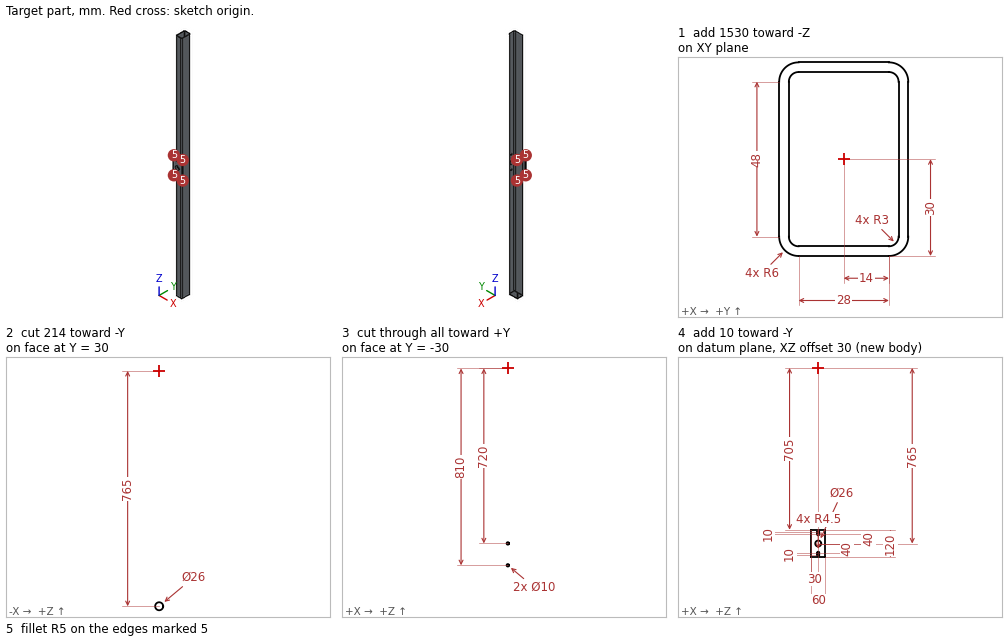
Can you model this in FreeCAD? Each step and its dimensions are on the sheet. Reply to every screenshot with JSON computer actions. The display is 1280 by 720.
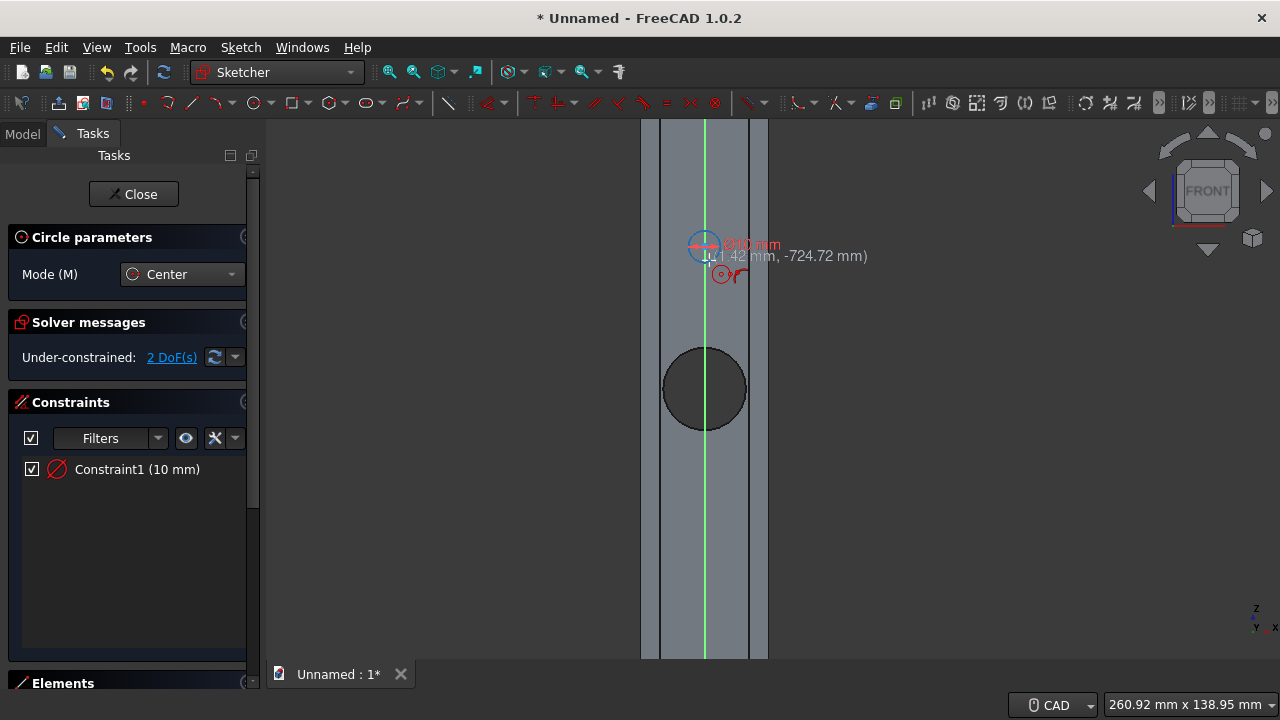
{"action": "scroll", "coordinate": [705, 532], "scroll_direction": "up", "scroll_amount": 2}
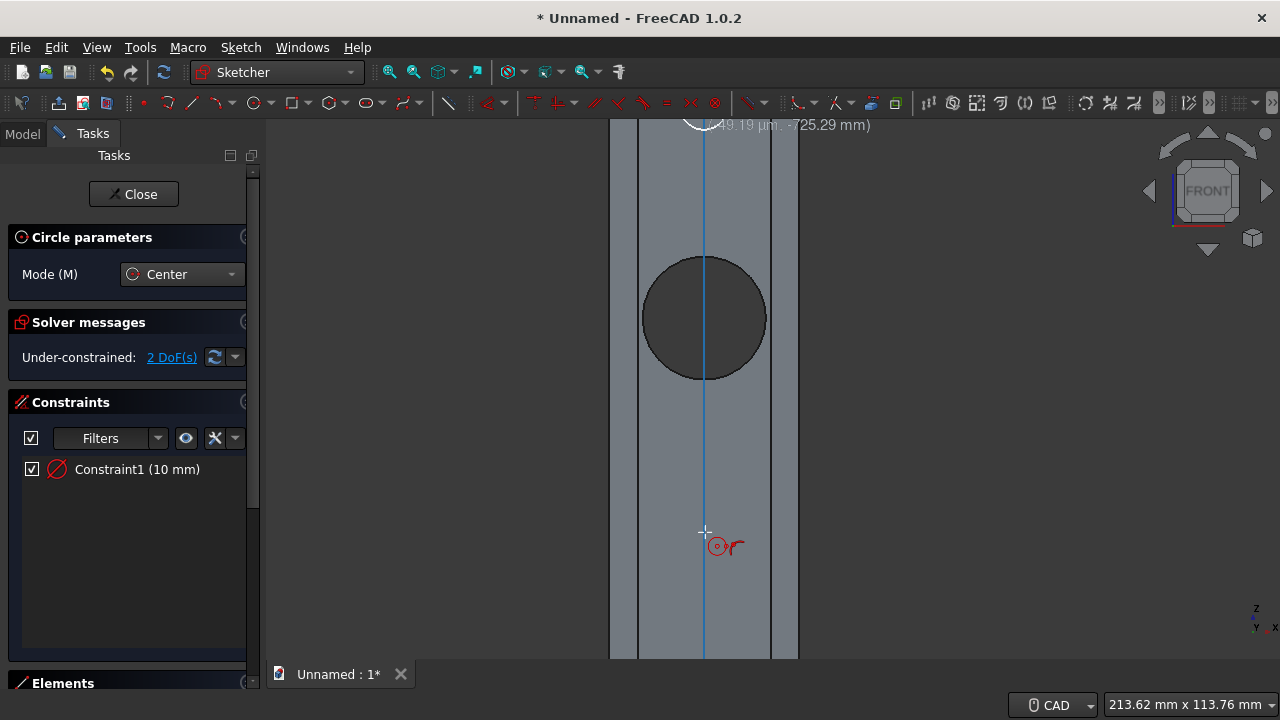
{"action": "left_click", "coordinate": [704, 532]}
{"action": "mouse_move", "coordinate": [721, 515]}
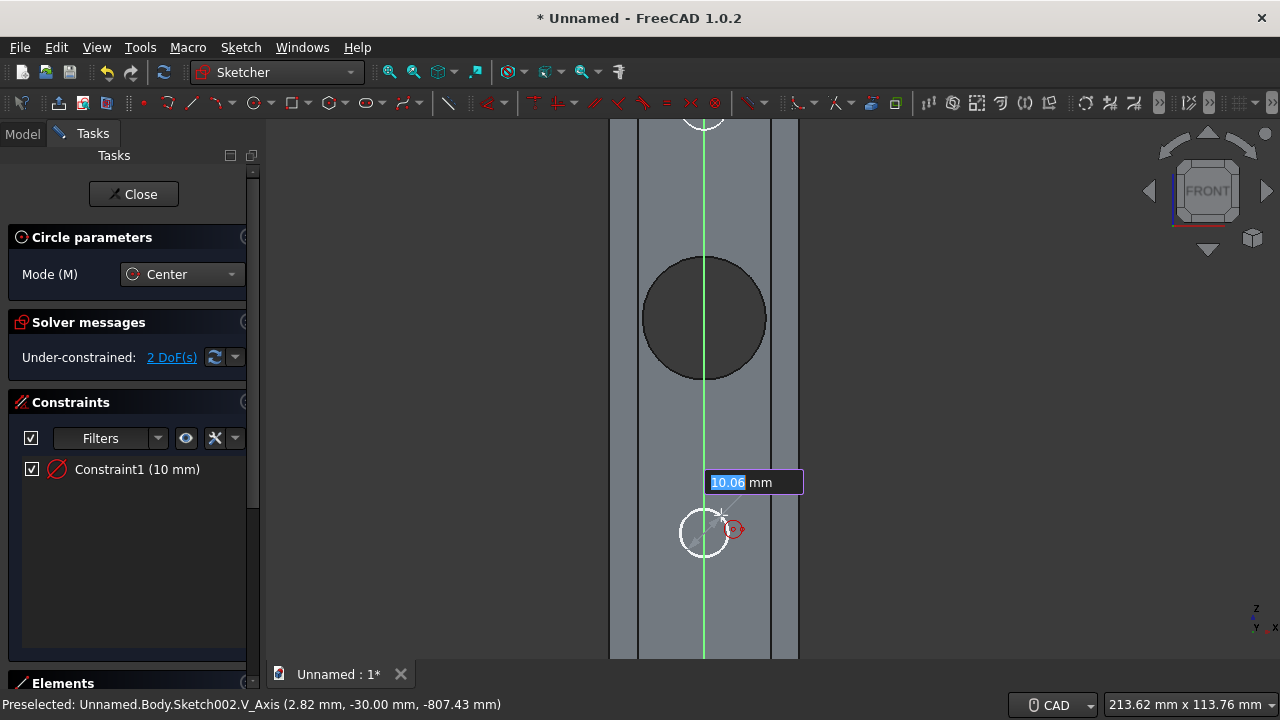
{"action": "type", "text": "10"}
{"action": "key", "text": "Return"}
{"action": "key", "text": "Escape"}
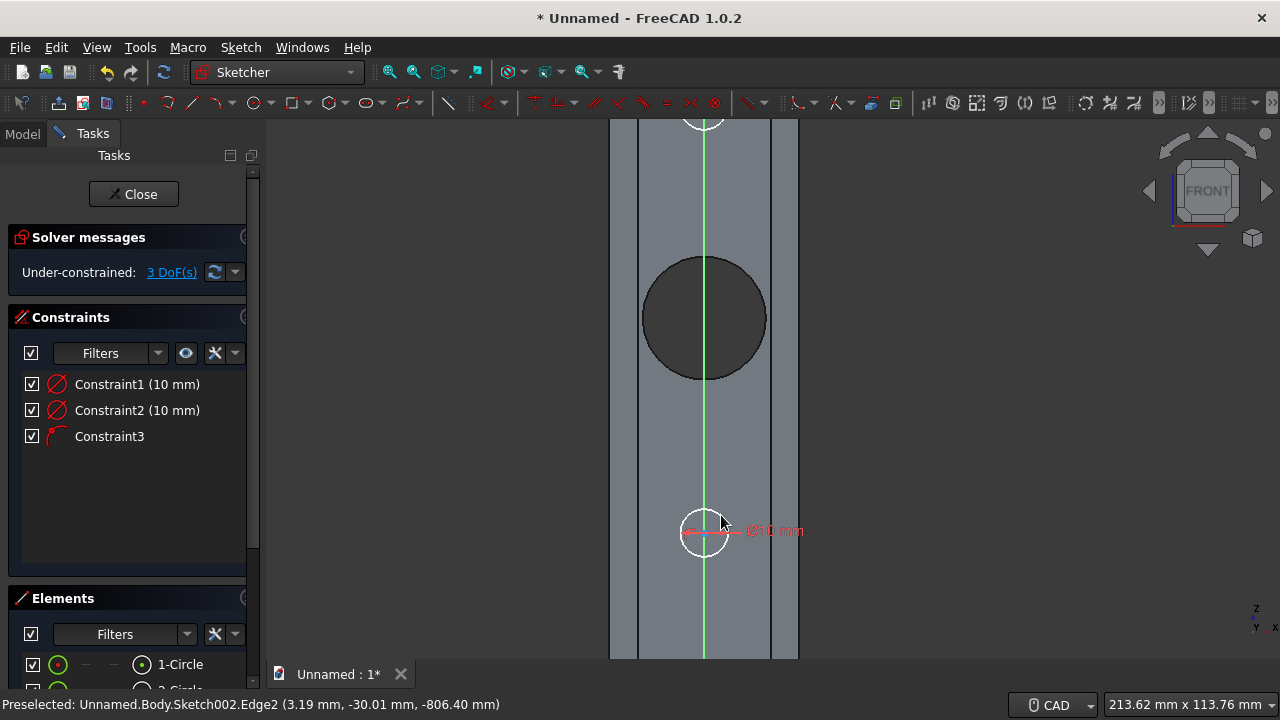
{"action": "scroll", "coordinate": [705, 533], "scroll_direction": "down", "scroll_amount": 2}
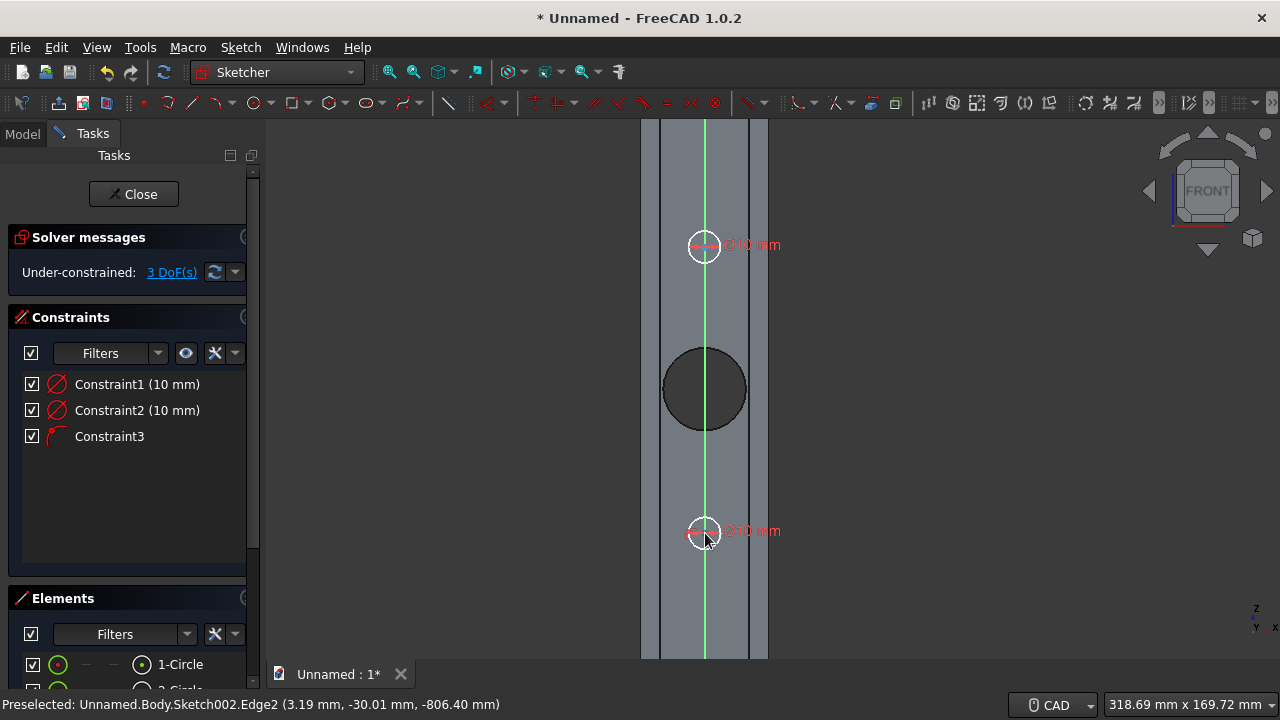
{"action": "left_click", "coordinate": [704, 247]}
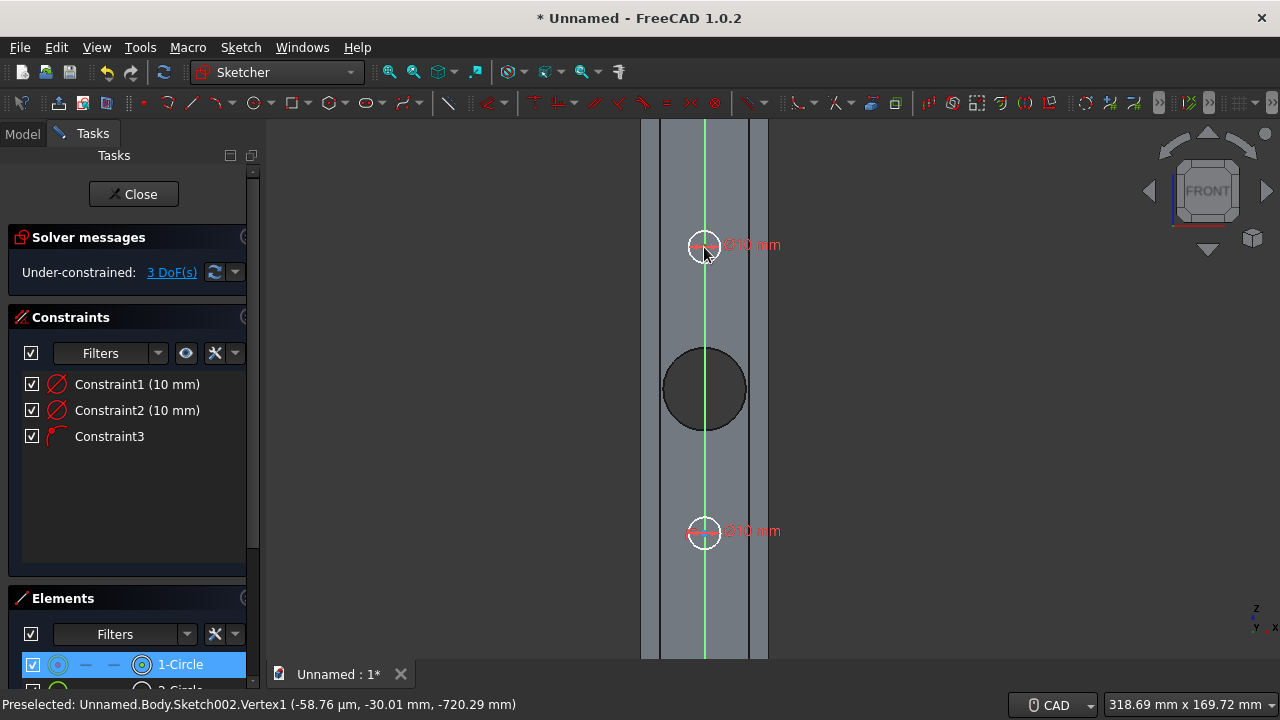
{"action": "left_click", "coordinate": [705, 596]}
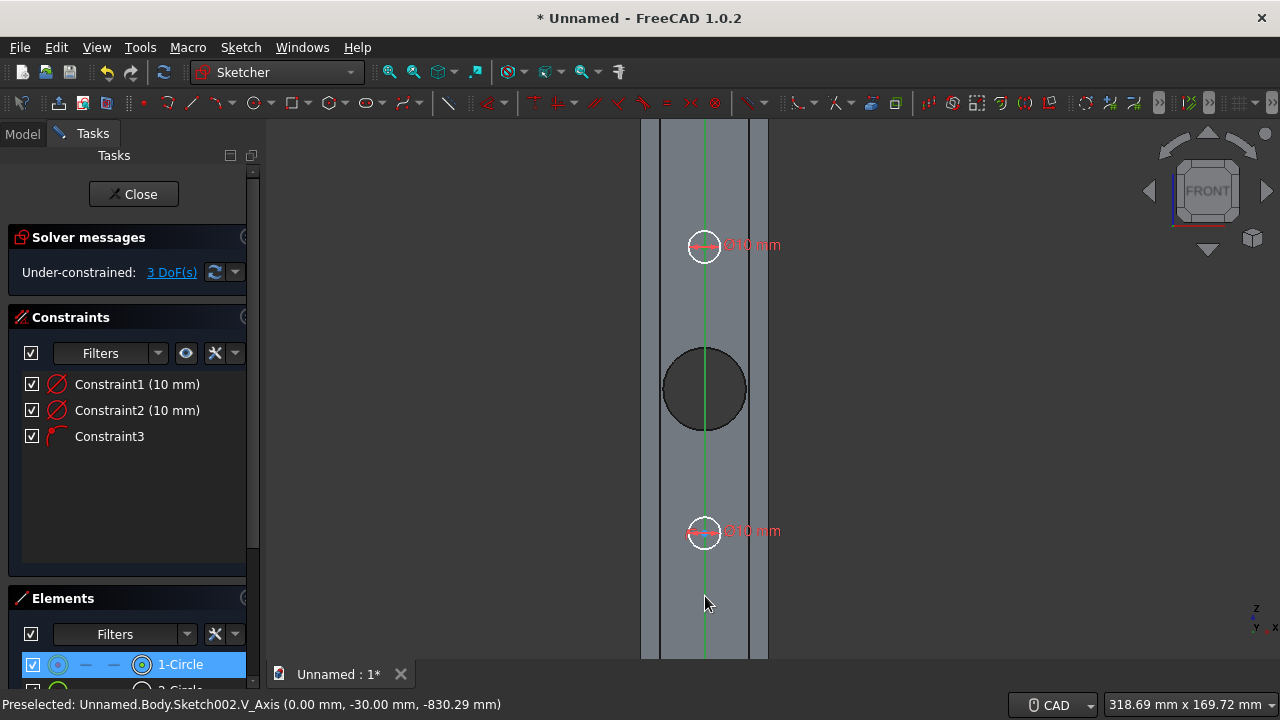
{"action": "left_click", "coordinate": [534, 104]}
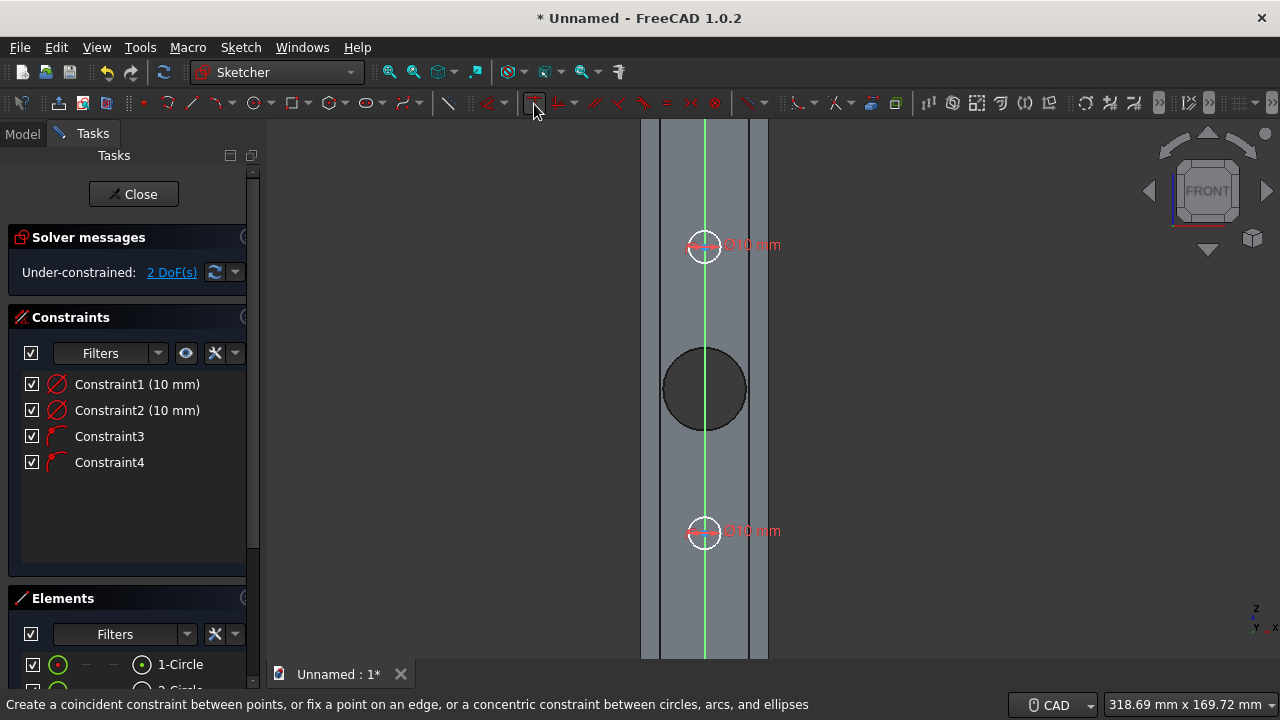
{"action": "left_click", "coordinate": [488, 104]}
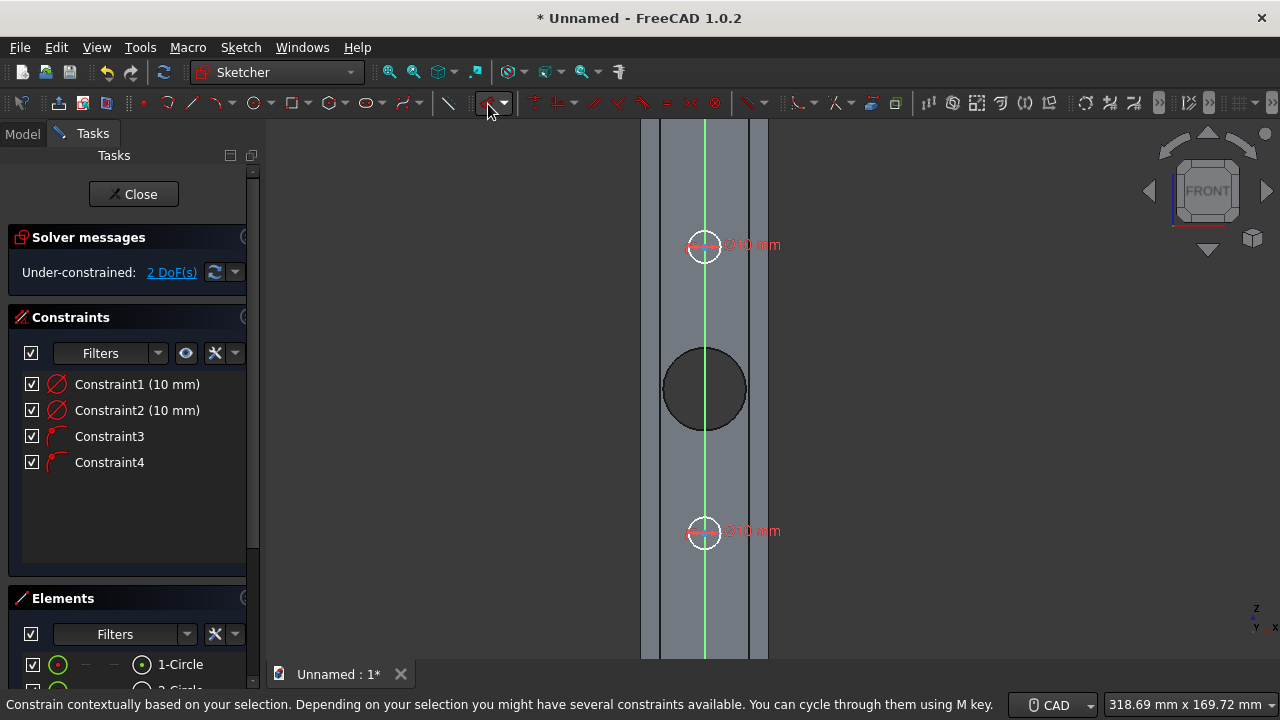
{"action": "left_click", "coordinate": [705, 247]}
{"action": "left_click", "coordinate": [739, 197]}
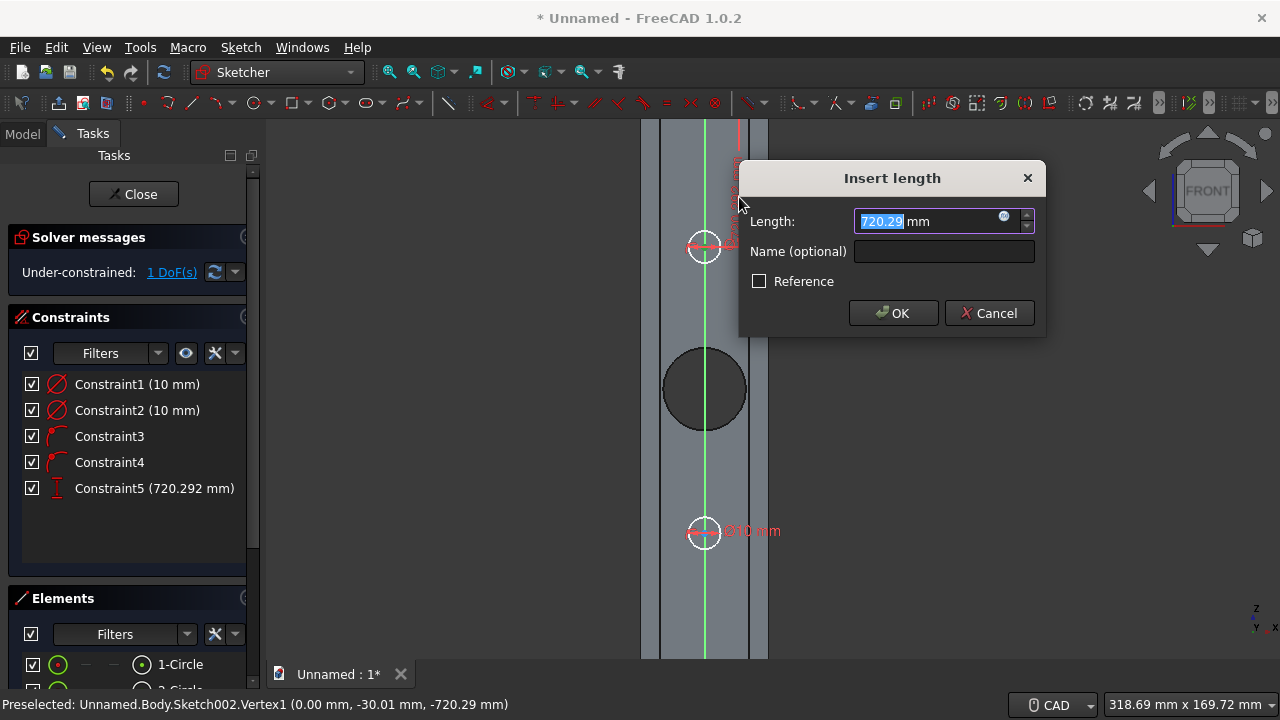
{"action": "type", "text": "720"}
{"action": "key", "text": "Return"}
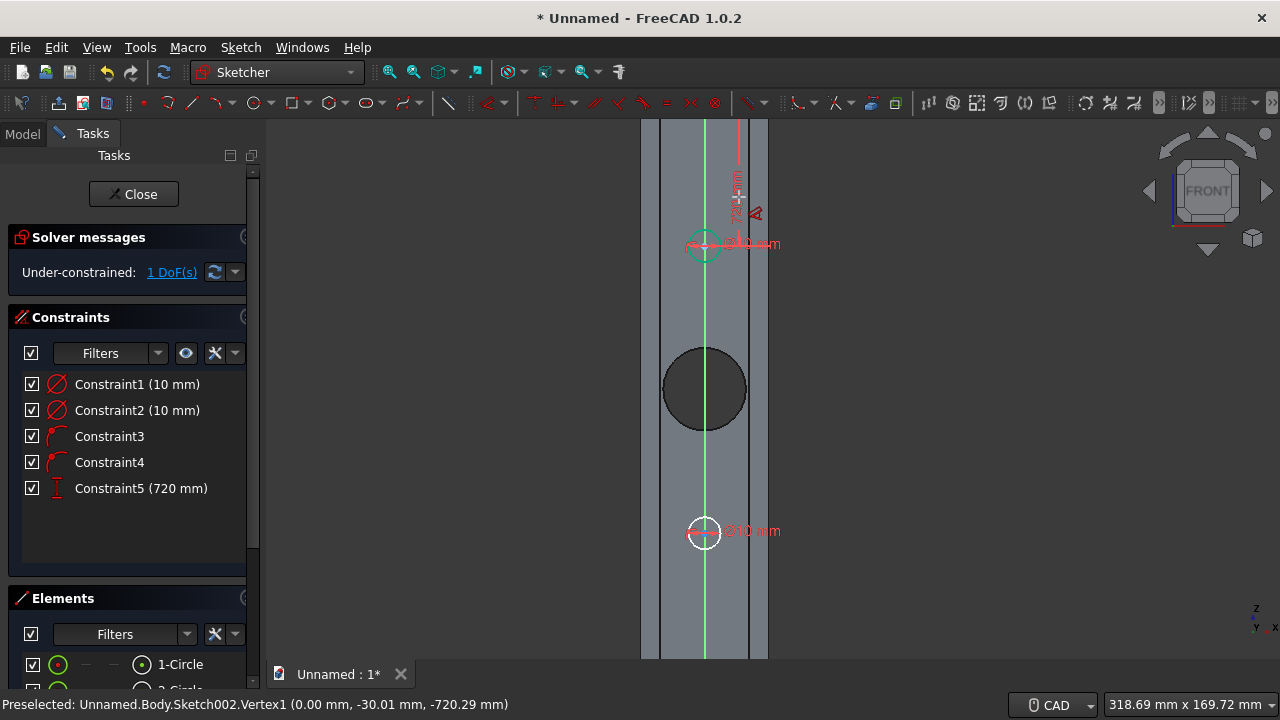
{"action": "left_click", "coordinate": [705, 533]}
{"action": "left_click", "coordinate": [739, 340]}